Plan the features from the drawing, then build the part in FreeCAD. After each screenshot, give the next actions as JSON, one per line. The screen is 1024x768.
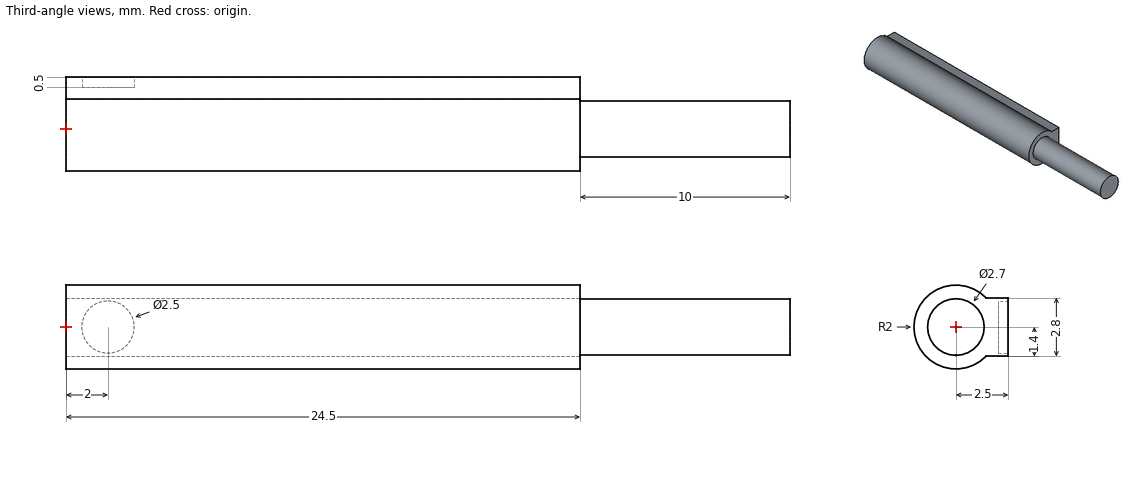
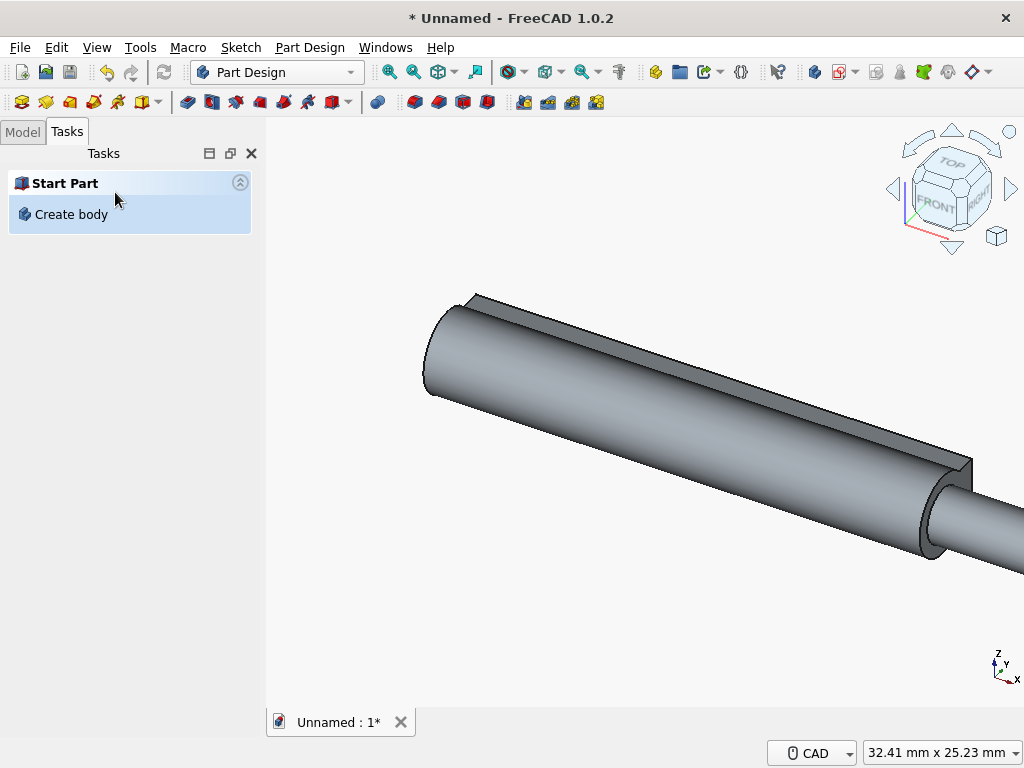
{"action": "key", "text": "v f"}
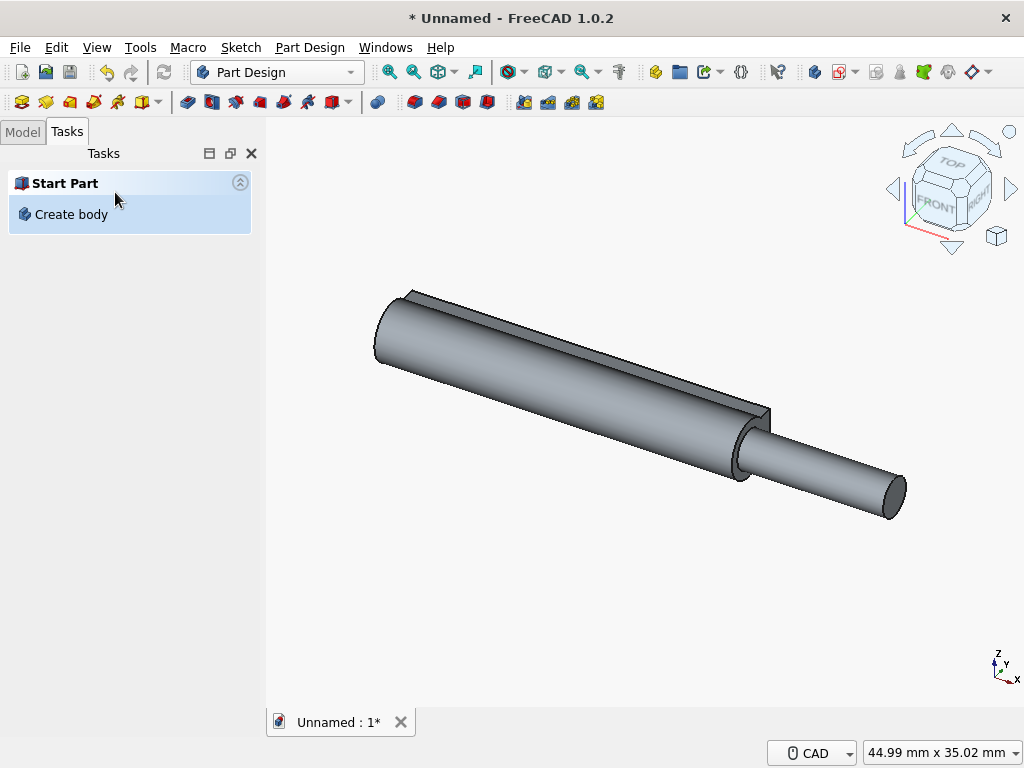
{"action": "key", "text": "4"}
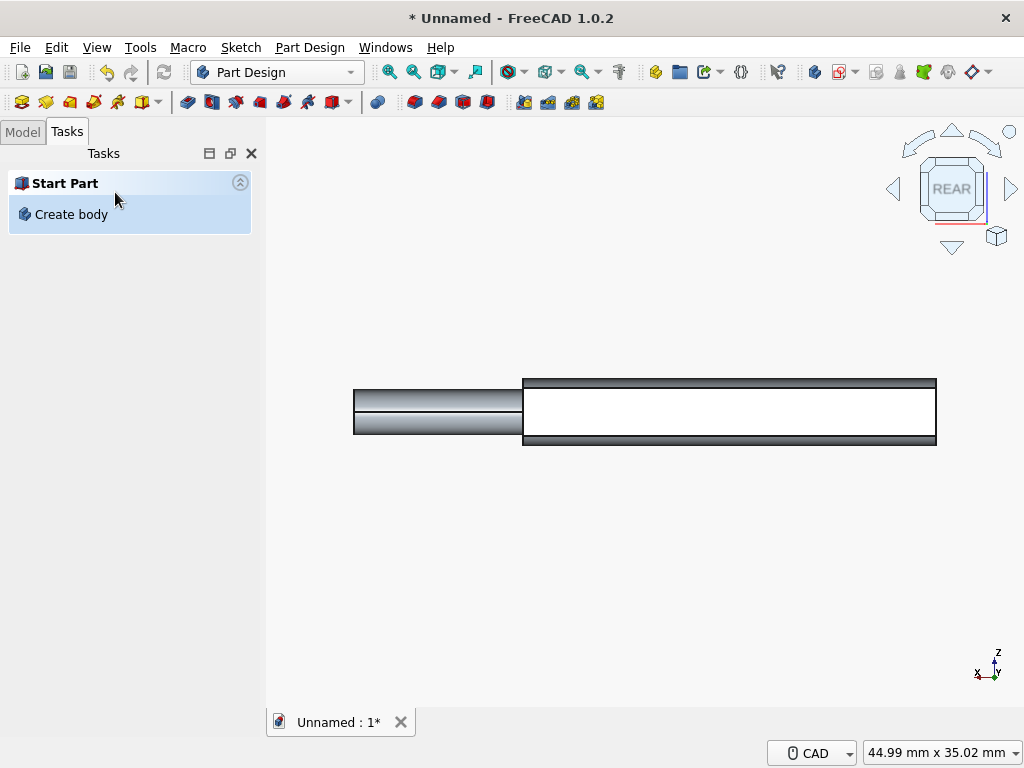
{"action": "left_click", "coordinate": [729, 411]}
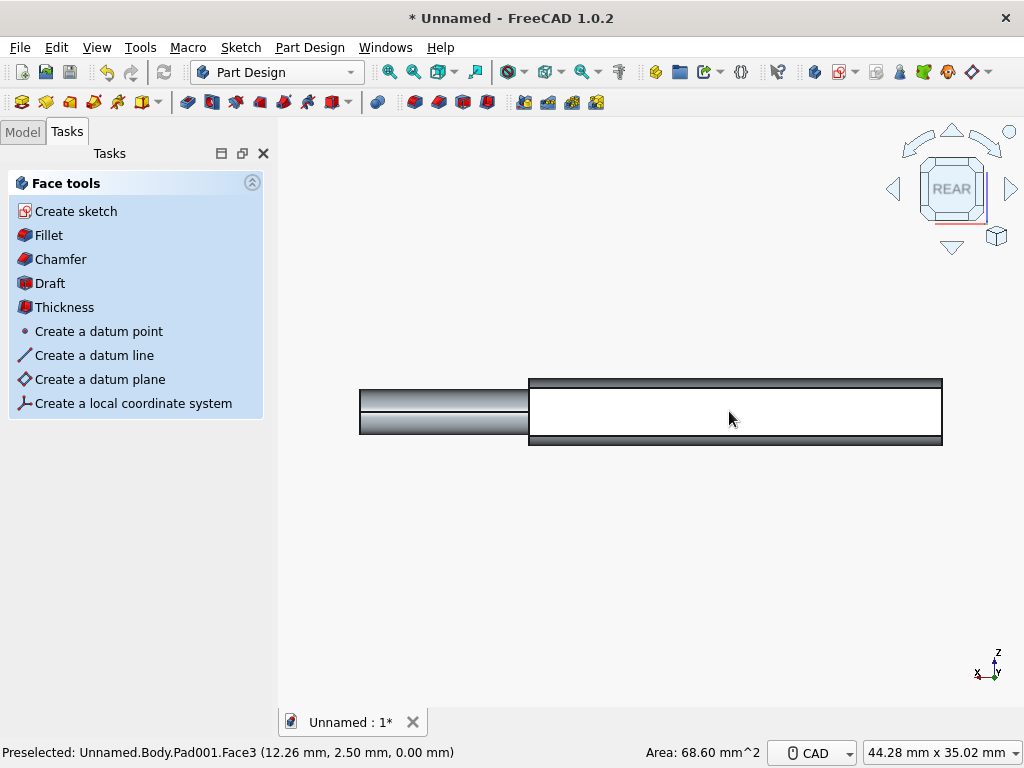
{"action": "left_click", "coordinate": [840, 72]}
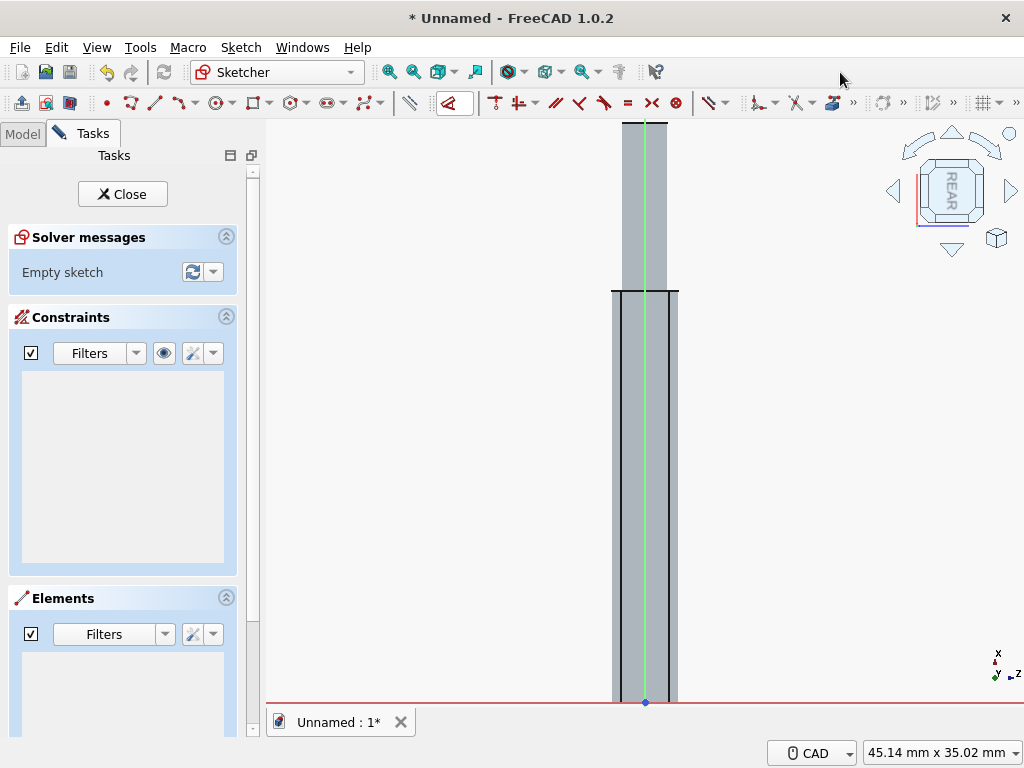
{"action": "scroll", "coordinate": [576, 413], "scroll_direction": "down", "scroll_amount": 5}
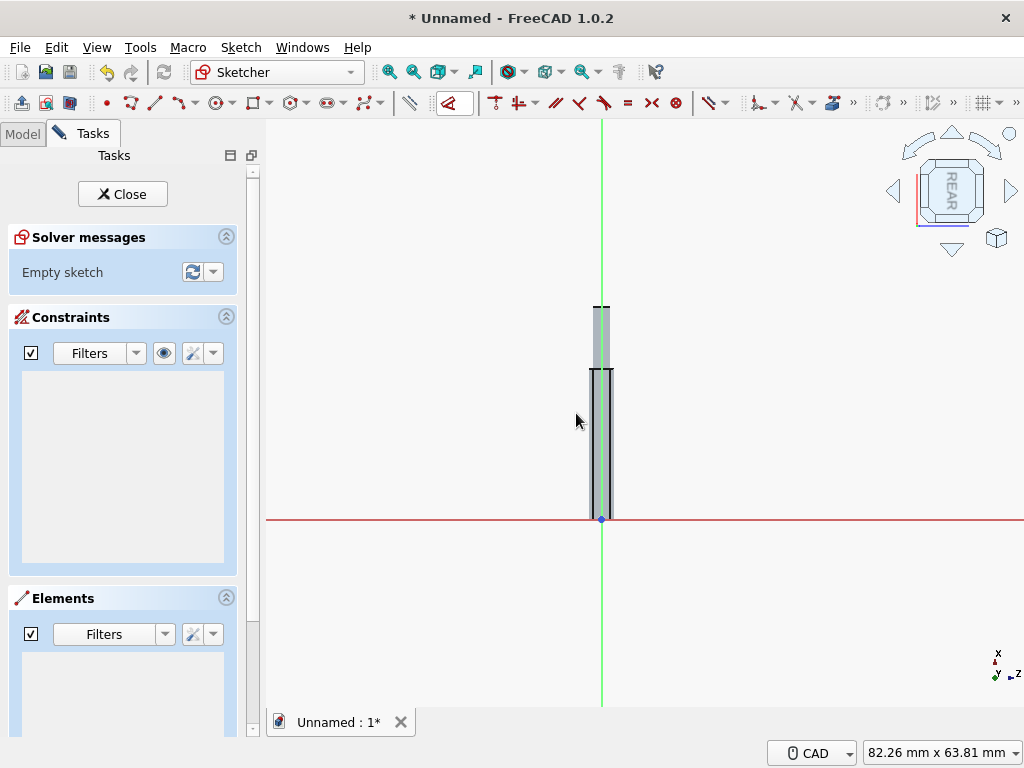
{"action": "scroll", "coordinate": [603, 515], "scroll_direction": "up", "scroll_amount": 15}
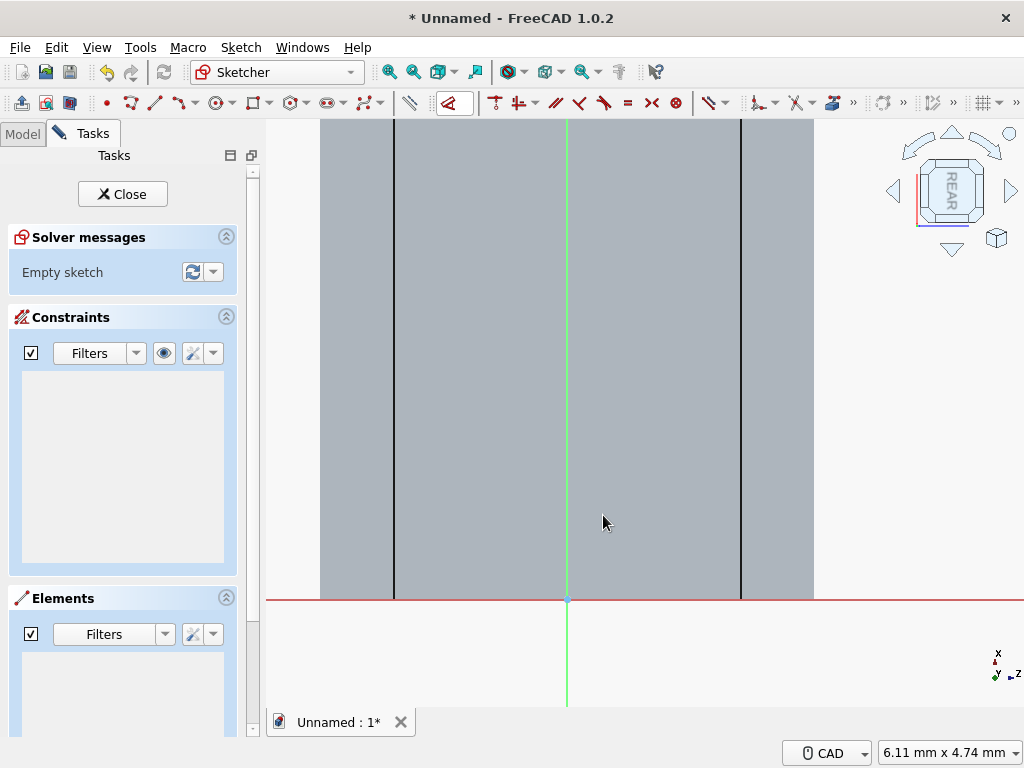
{"action": "left_click", "coordinate": [216, 104]}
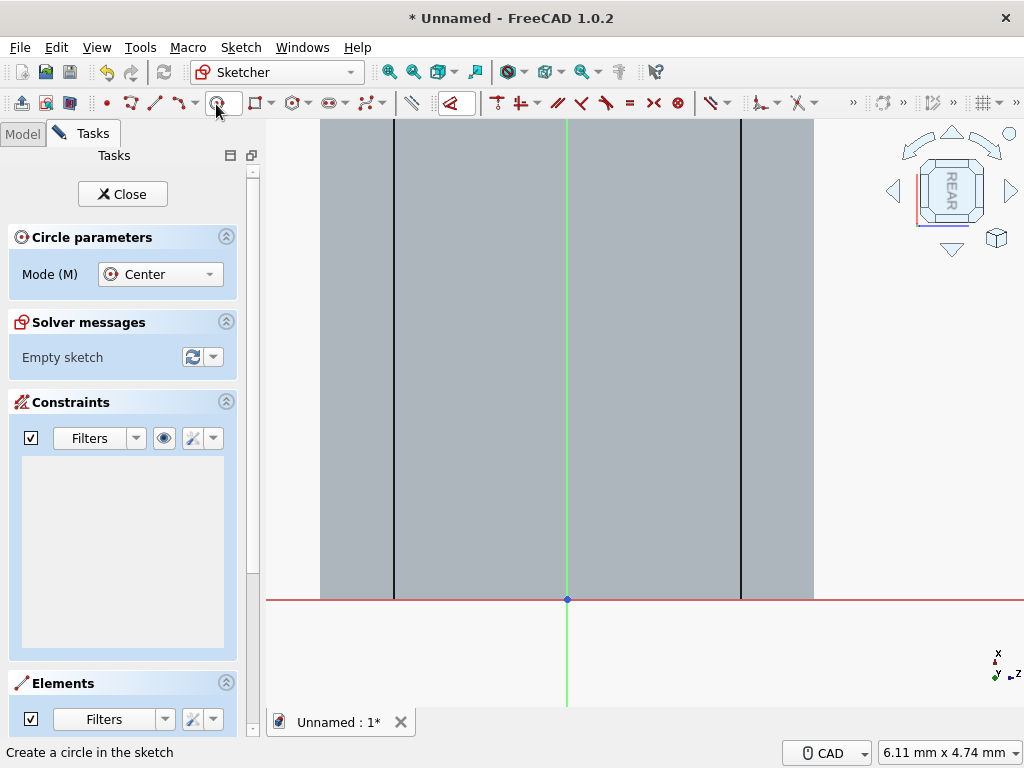
{"action": "left_click", "coordinate": [567, 352]}
{"action": "mouse_move", "coordinate": [677, 242]}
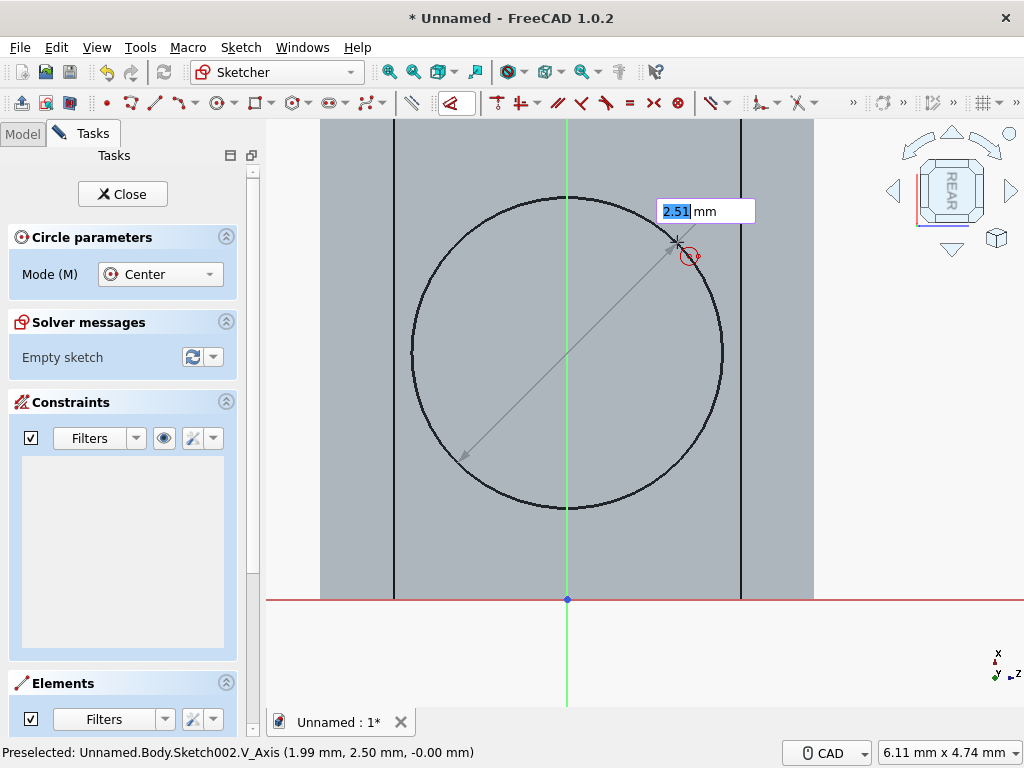
{"action": "type", "text": "2.5"}
{"action": "key", "text": "Return"}
{"action": "key", "text": "Escape"}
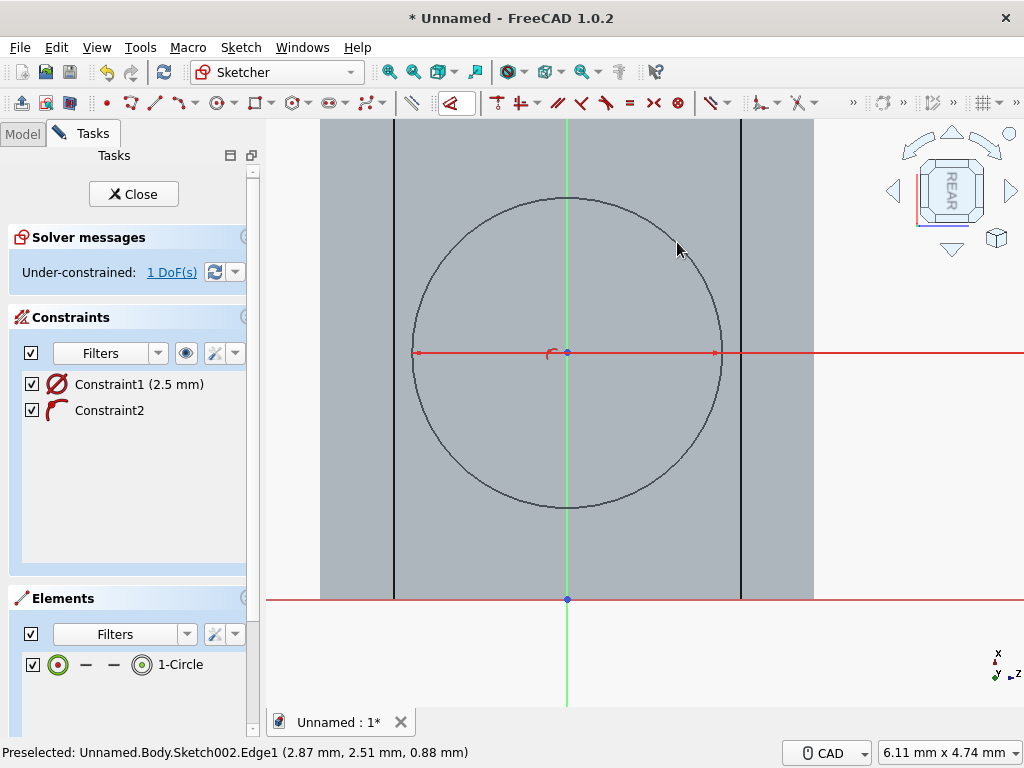
{"action": "left_click", "coordinate": [567, 353]}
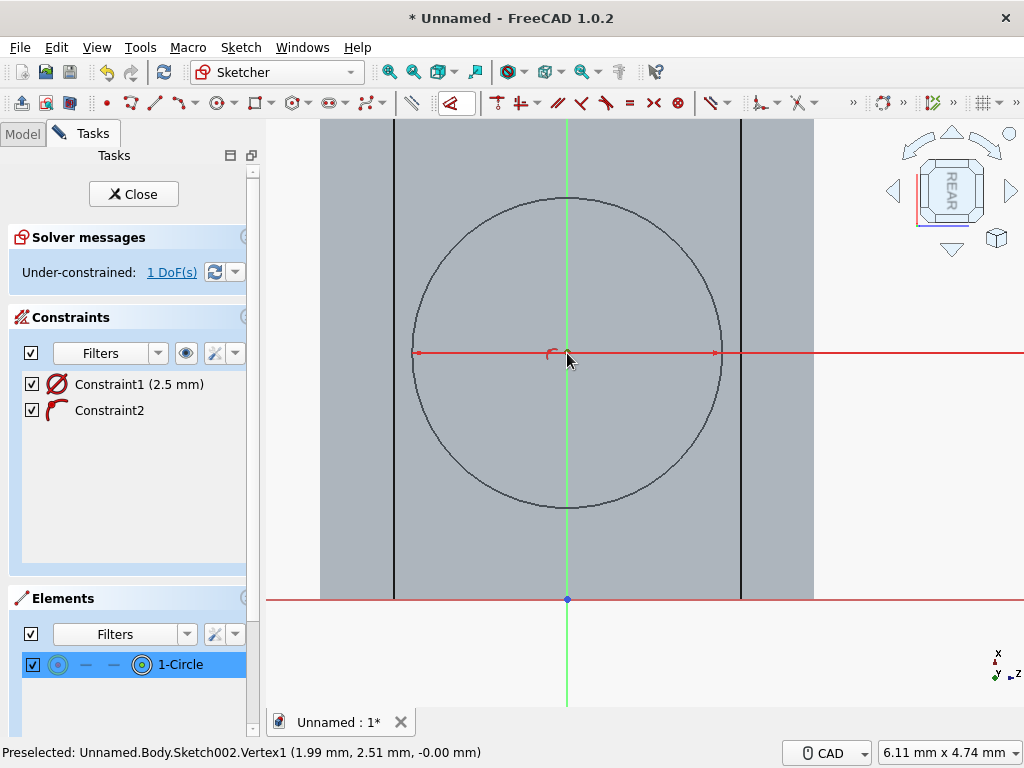
{"action": "key", "text": "i"}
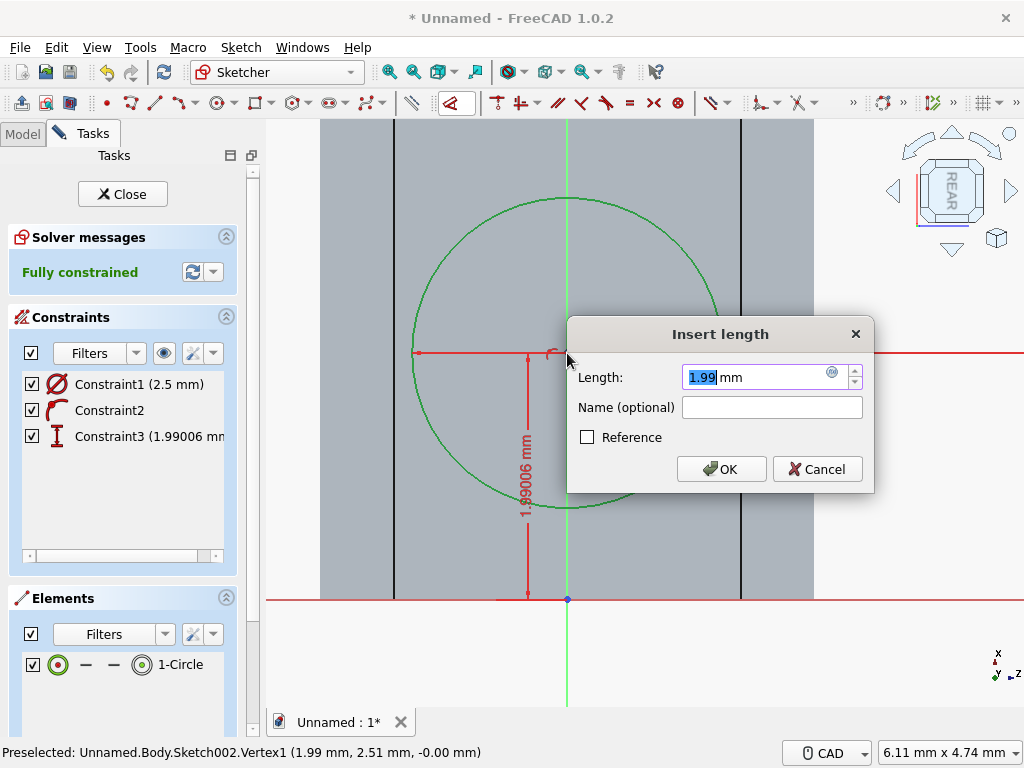
{"action": "type", "text": "2"}
{"action": "key", "text": "Return"}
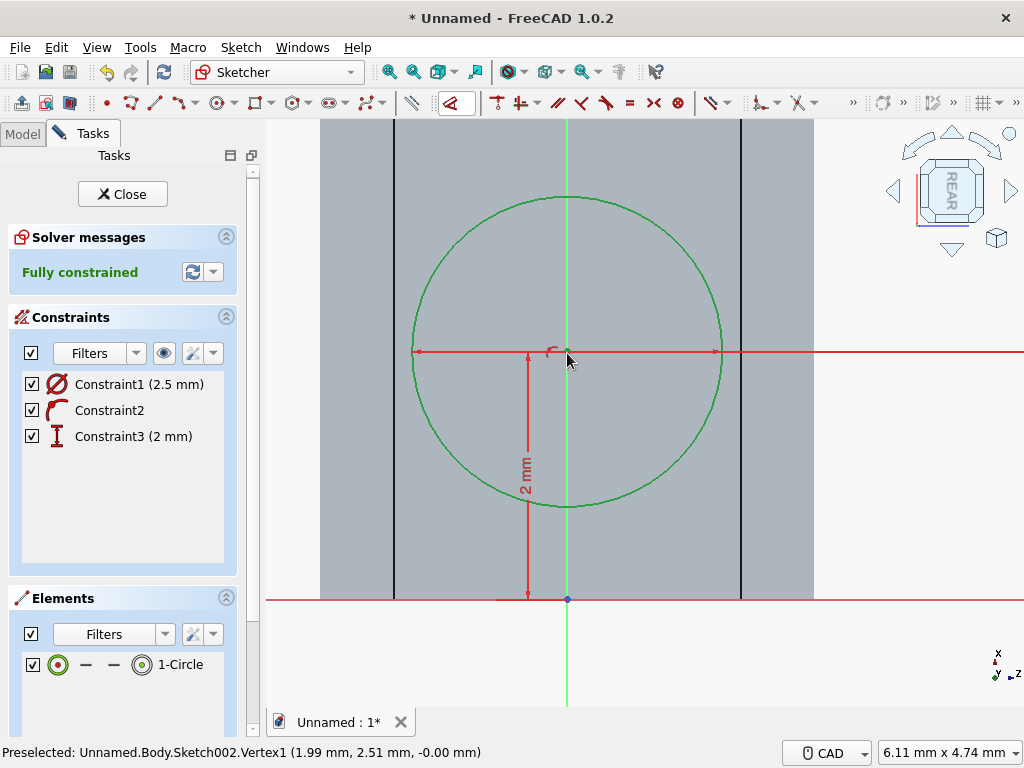
{"action": "left_click", "coordinate": [123, 194]}